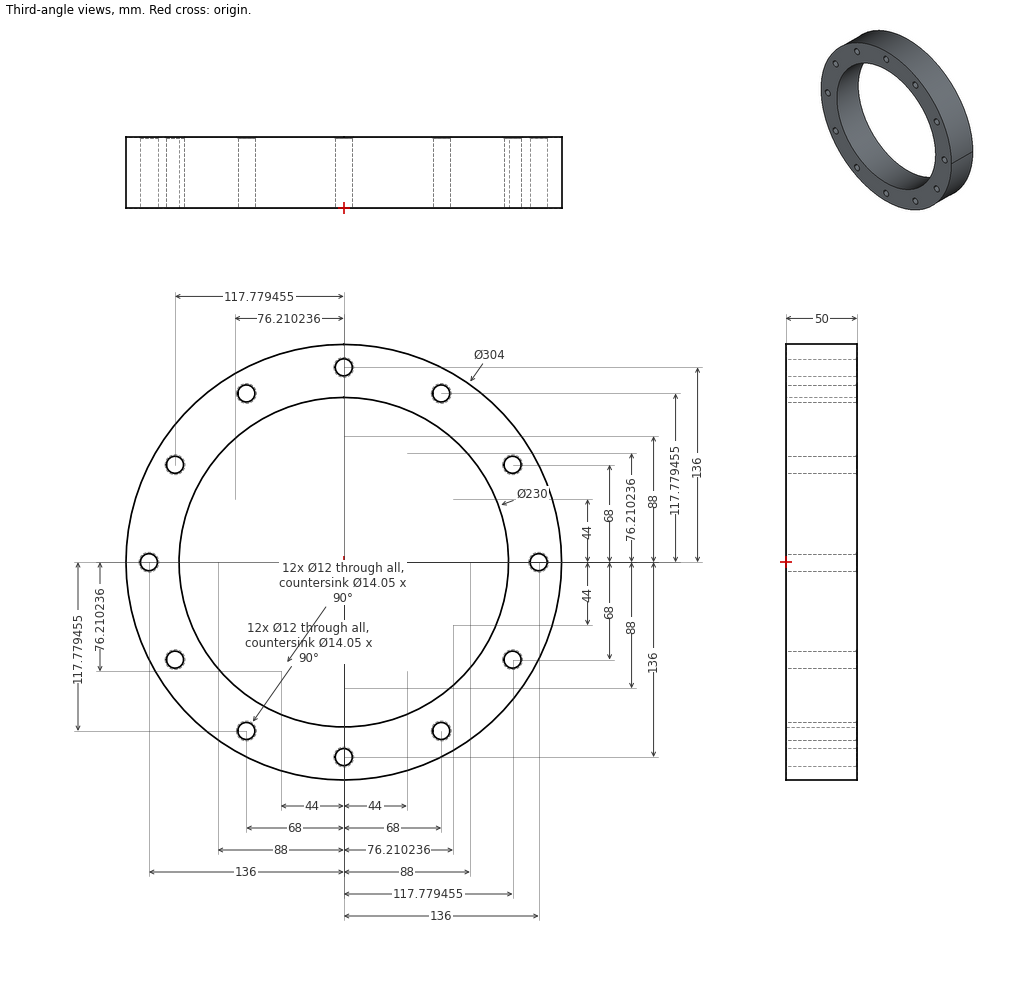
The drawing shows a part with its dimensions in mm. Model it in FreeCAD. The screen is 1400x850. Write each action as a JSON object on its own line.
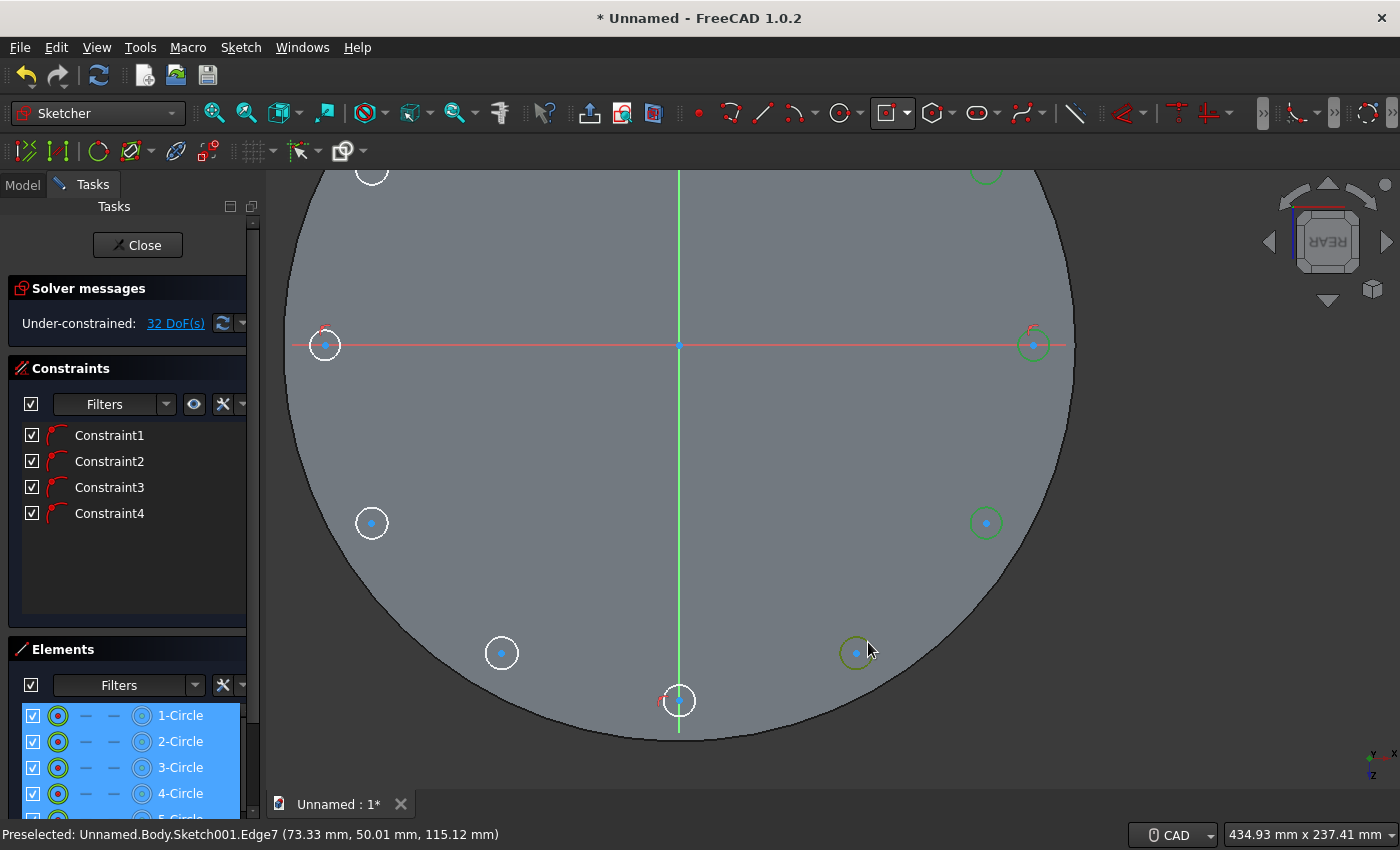
{"action": "scroll", "coordinate": [690, 690], "scroll_direction": "up", "scroll_amount": 2}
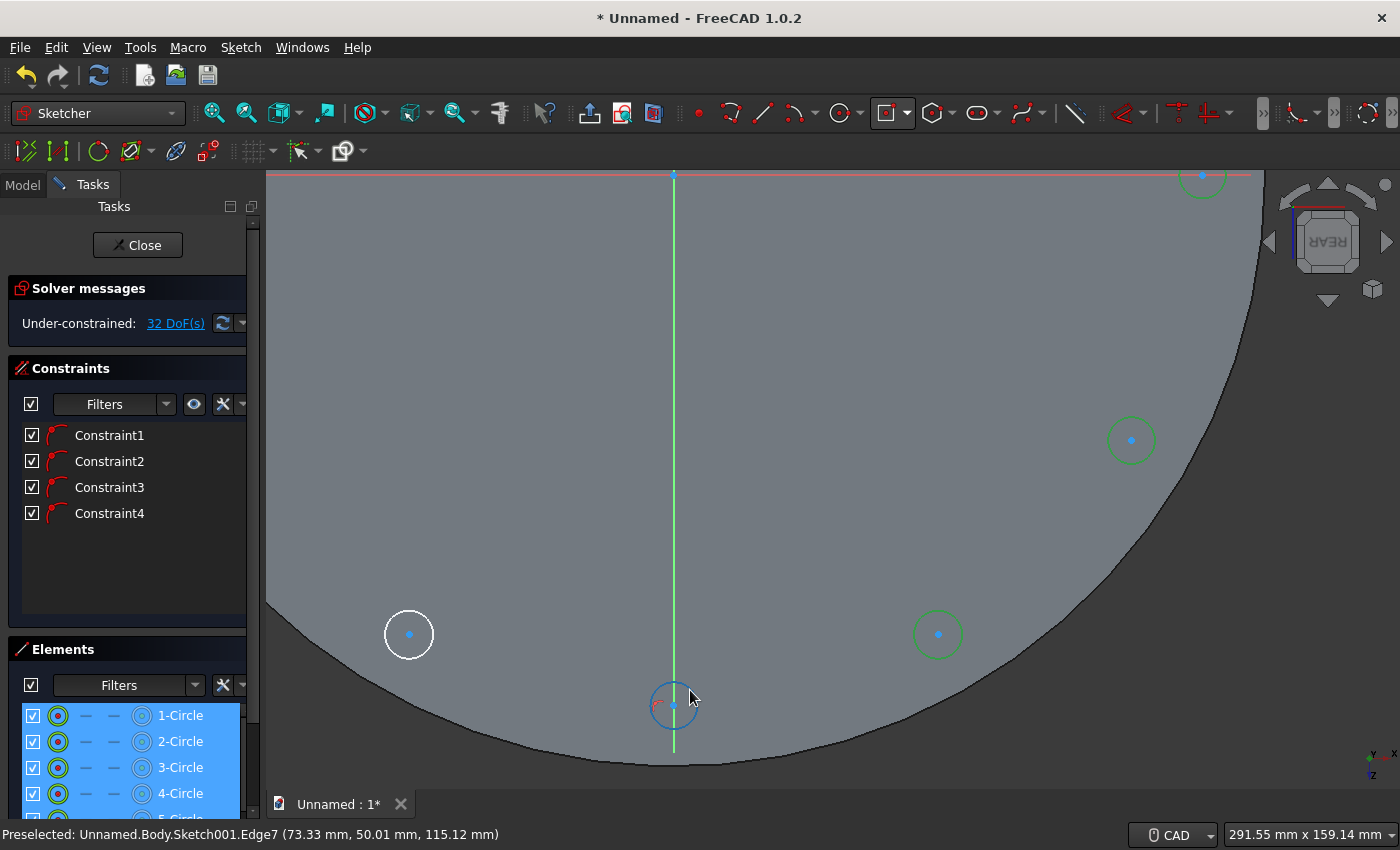
{"action": "left_click", "coordinate": [690, 689]}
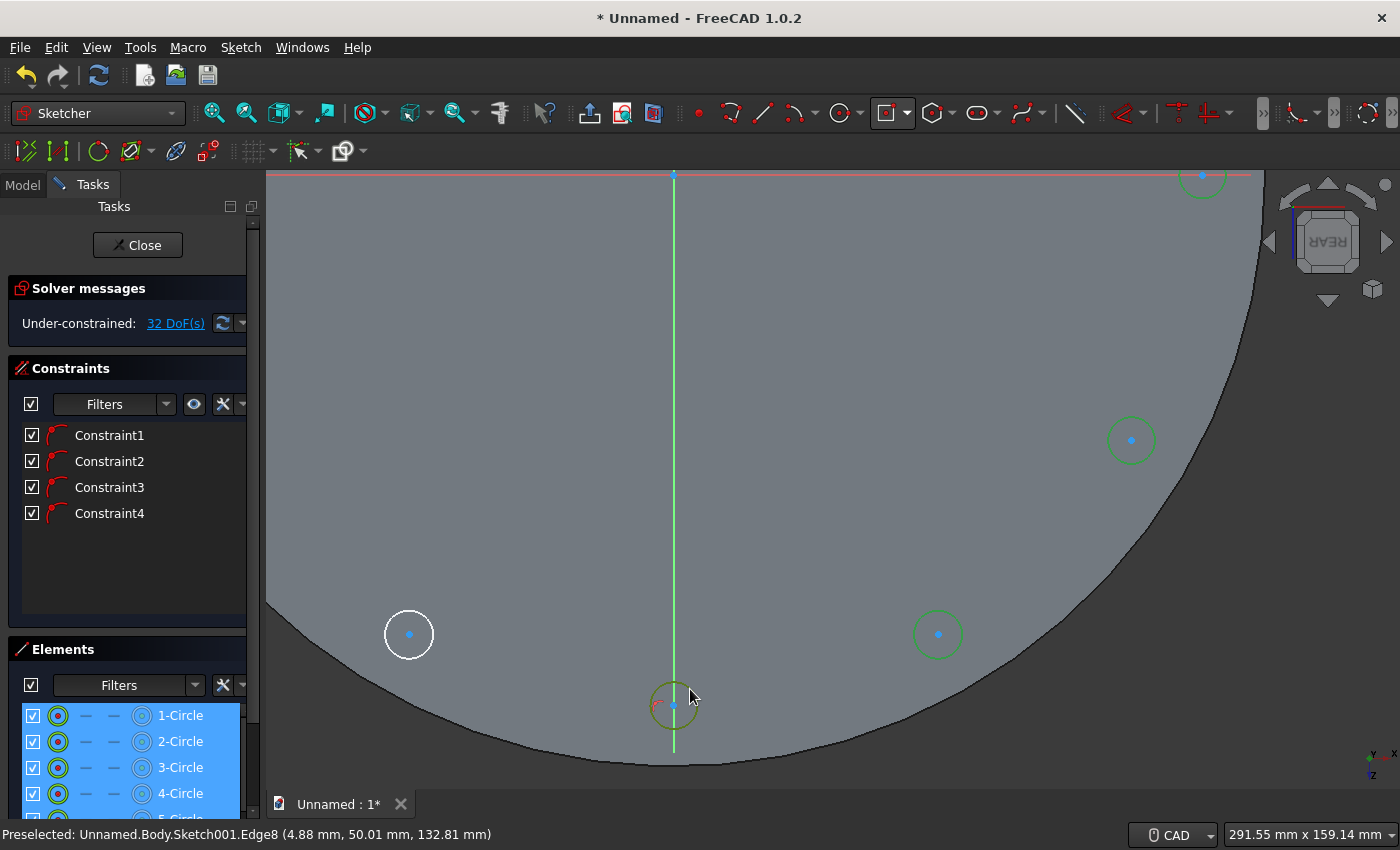
{"action": "left_click", "coordinate": [426, 618]}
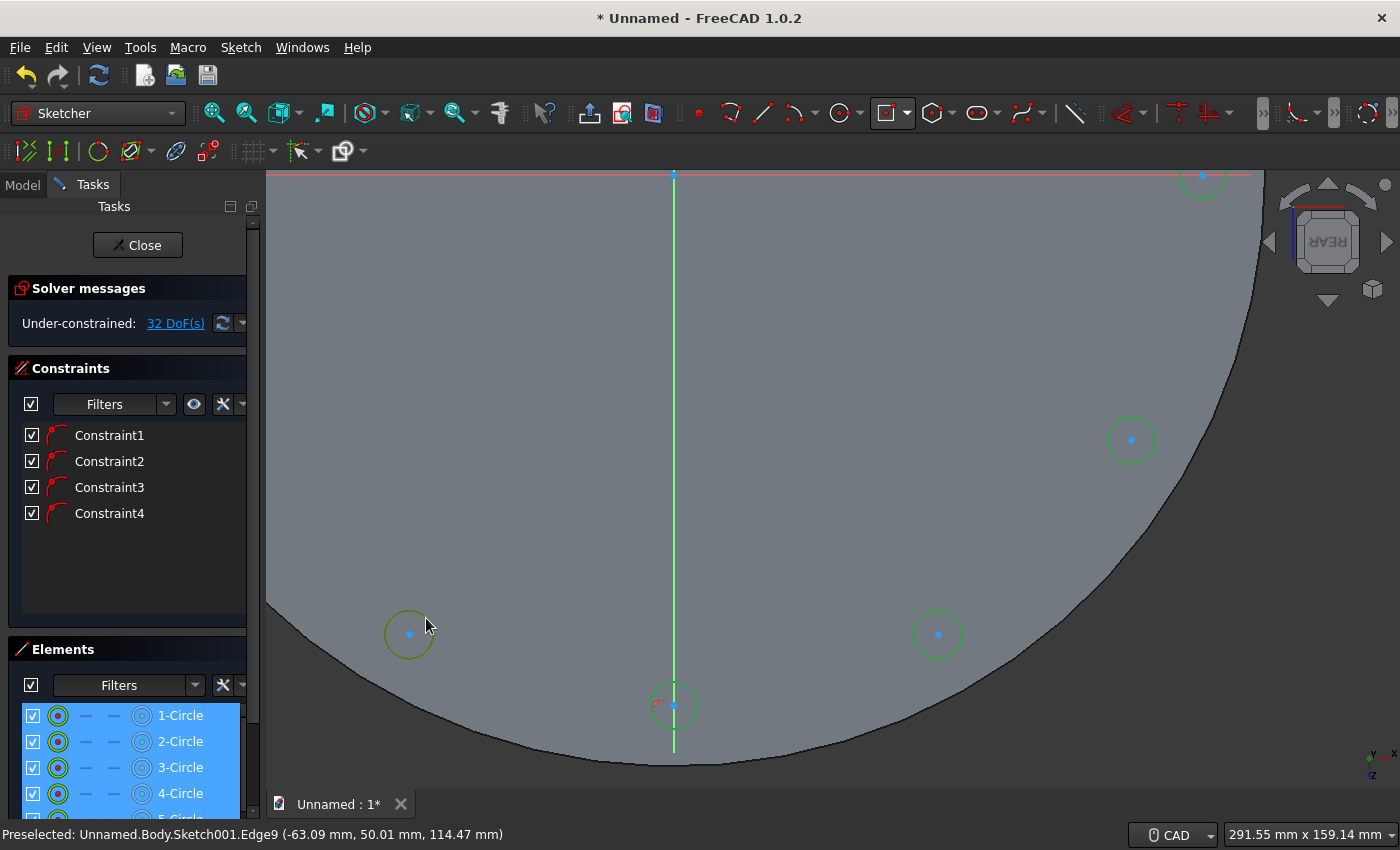
{"action": "scroll", "coordinate": [817, 657], "scroll_direction": "down", "scroll_amount": 5}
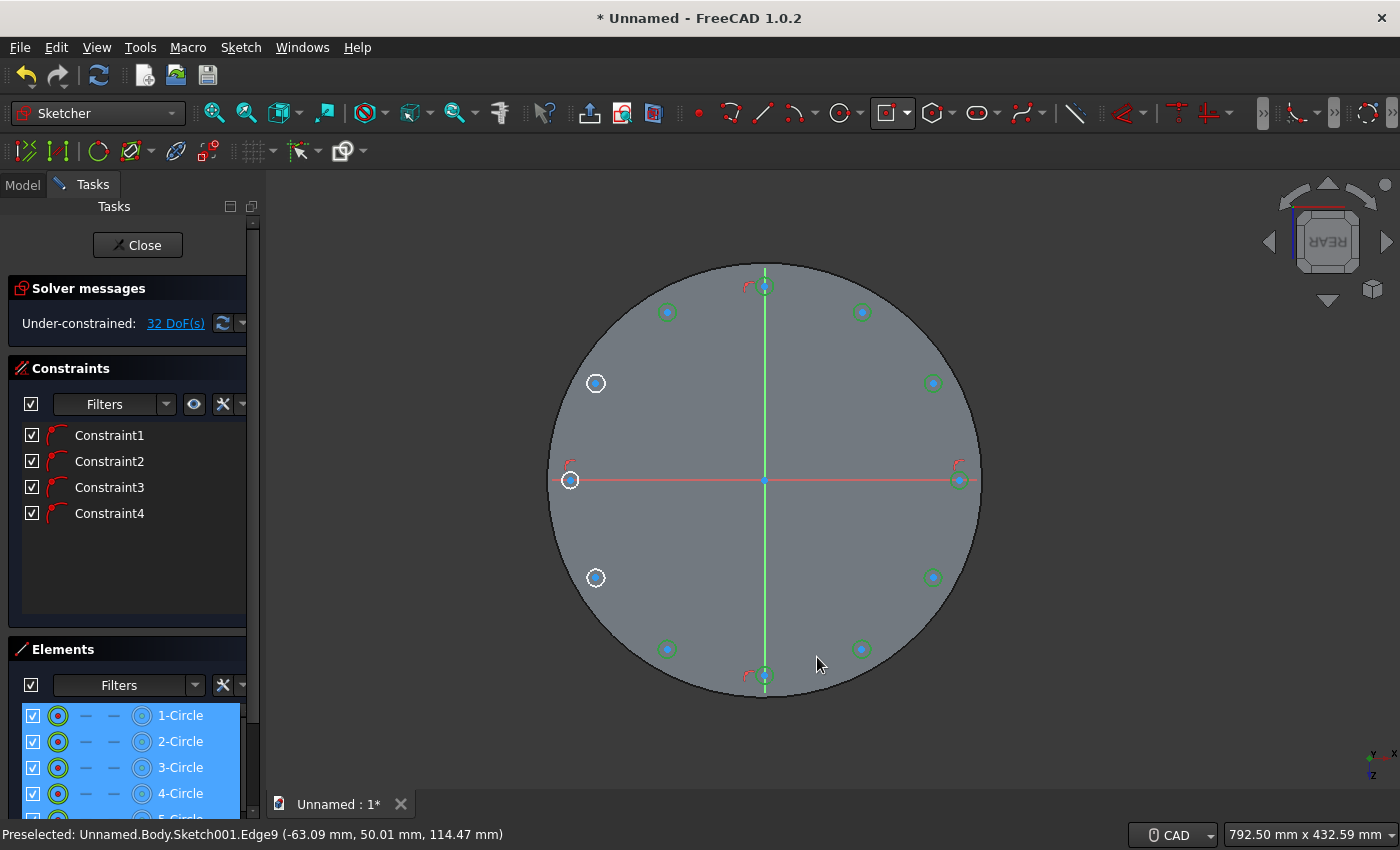
{"action": "scroll", "coordinate": [602, 572], "scroll_direction": "up", "scroll_amount": 3}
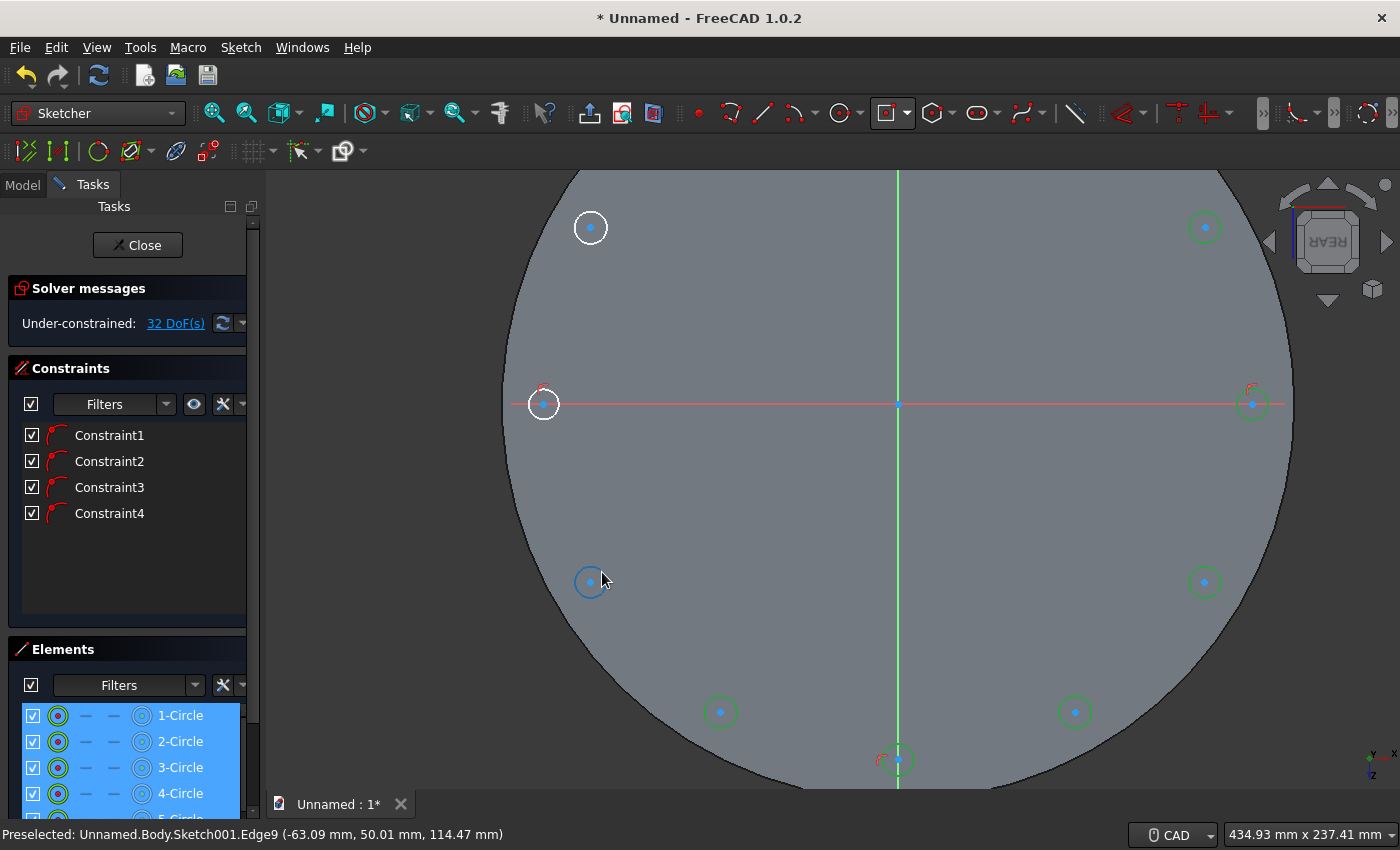
{"action": "left_click", "coordinate": [602, 571]}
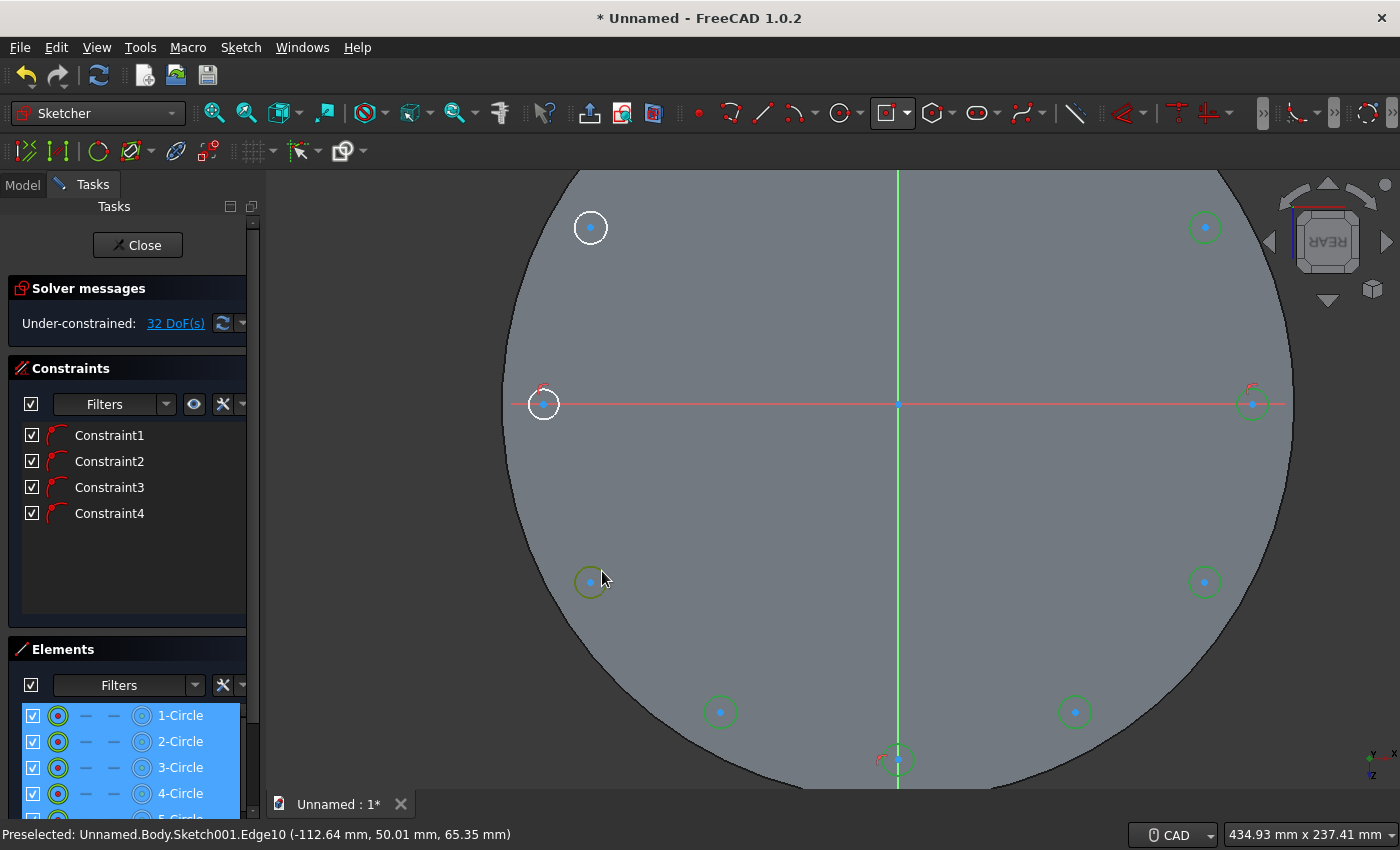
{"action": "scroll", "coordinate": [554, 394], "scroll_direction": "up", "scroll_amount": 2}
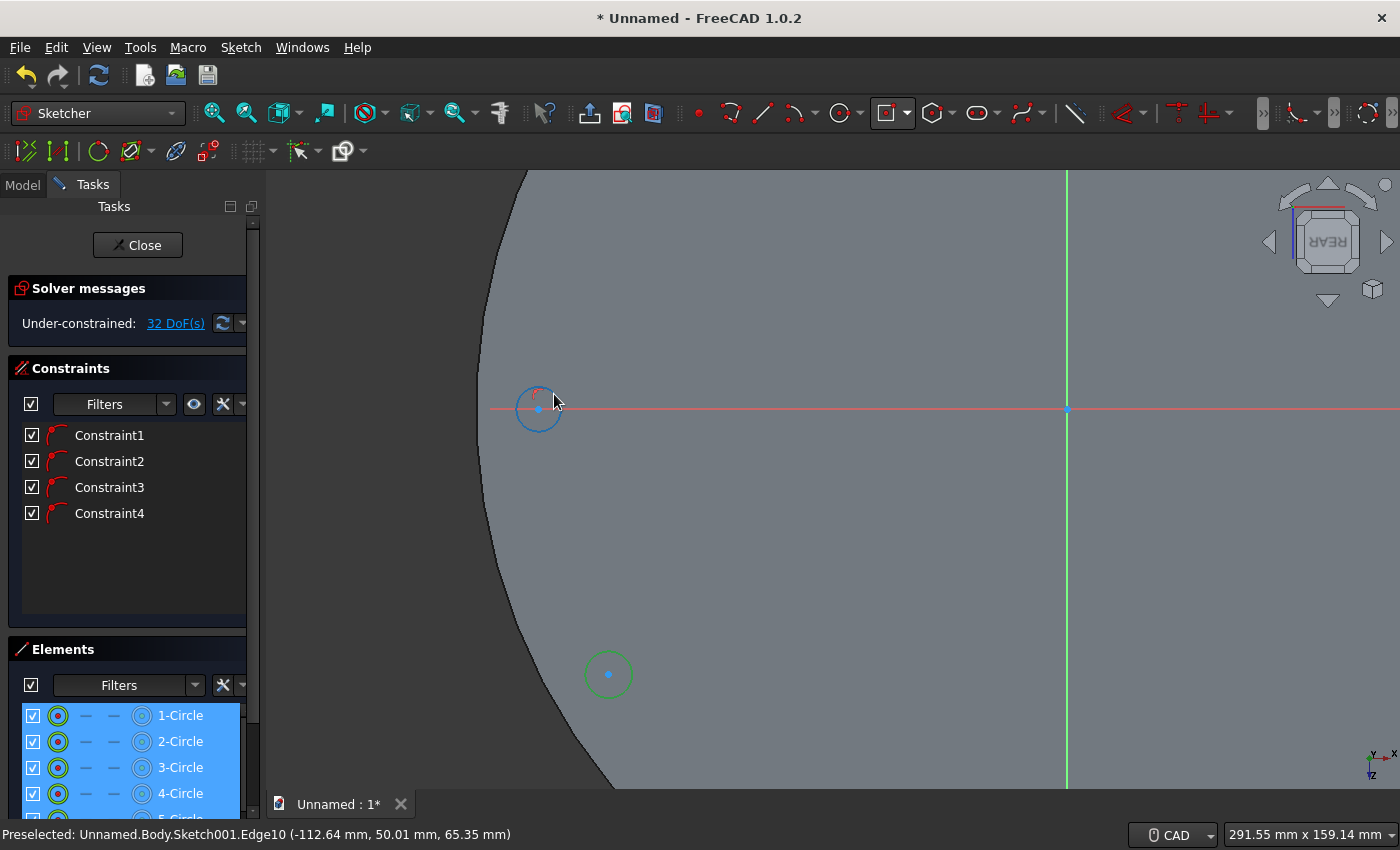
{"action": "left_click", "coordinate": [554, 393]}